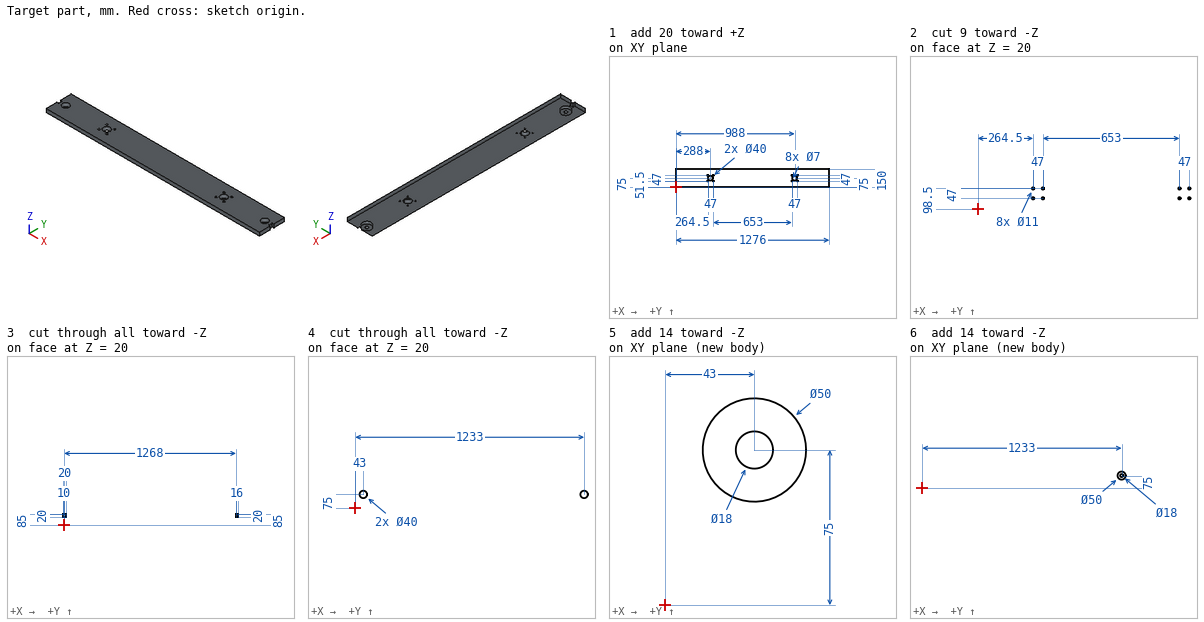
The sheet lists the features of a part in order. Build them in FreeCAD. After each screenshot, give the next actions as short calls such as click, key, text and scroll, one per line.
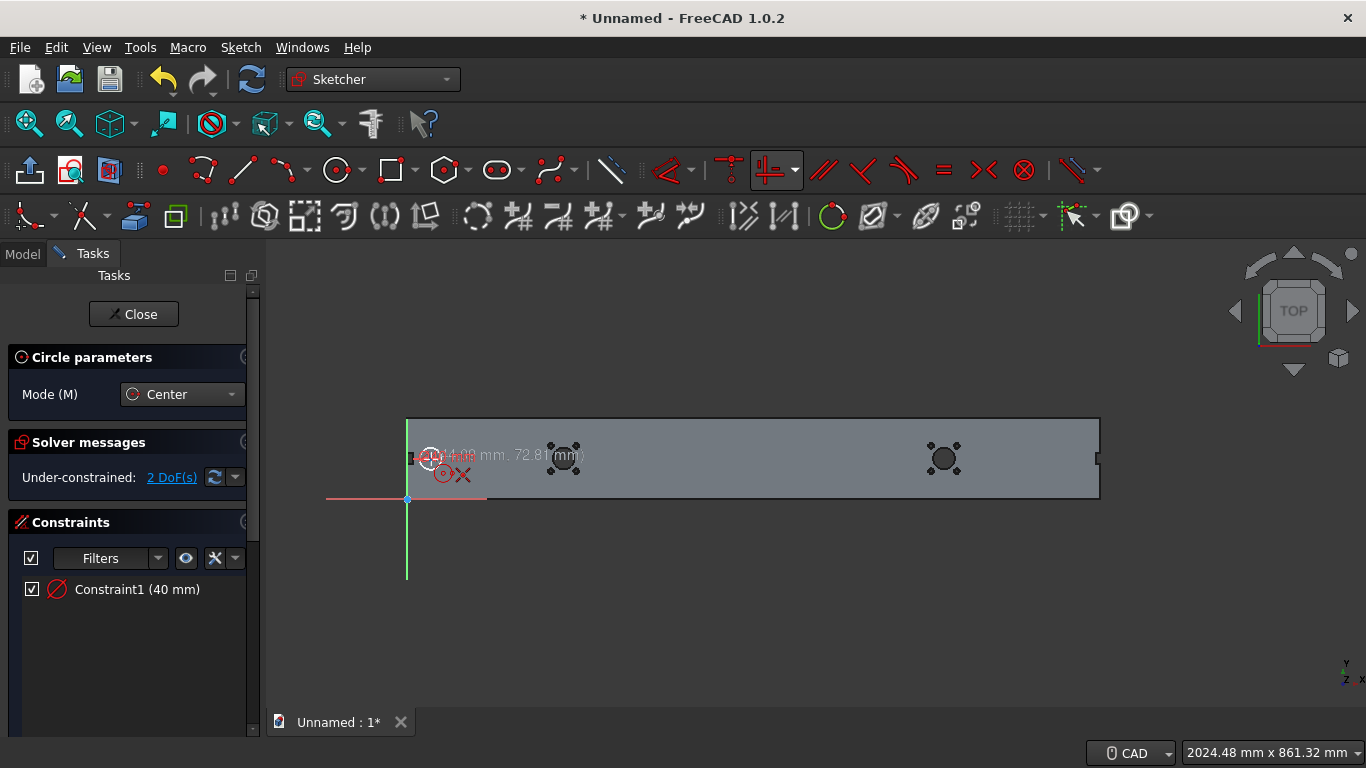
scroll(1077, 459, up, 4)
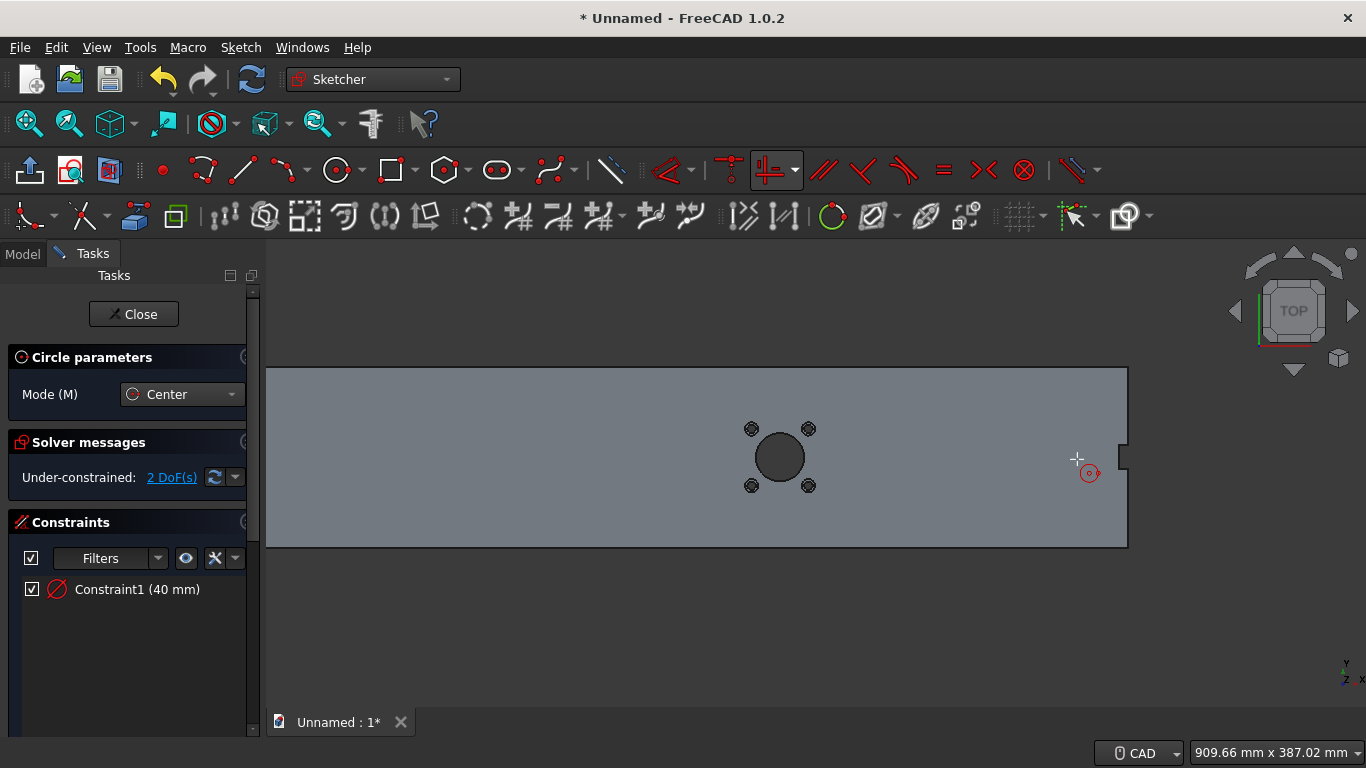
click(1076, 457)
move(1093, 440)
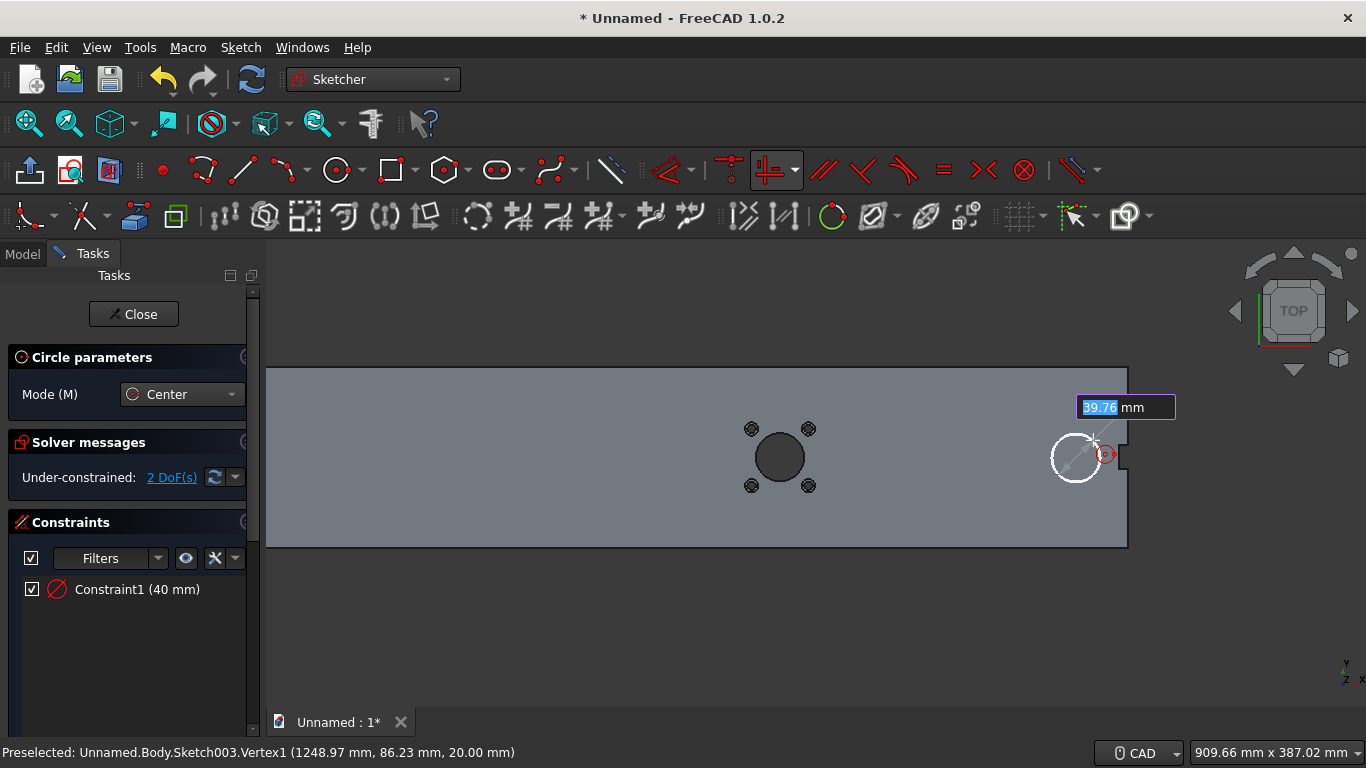
text(40)
key(Return)
key(Escape)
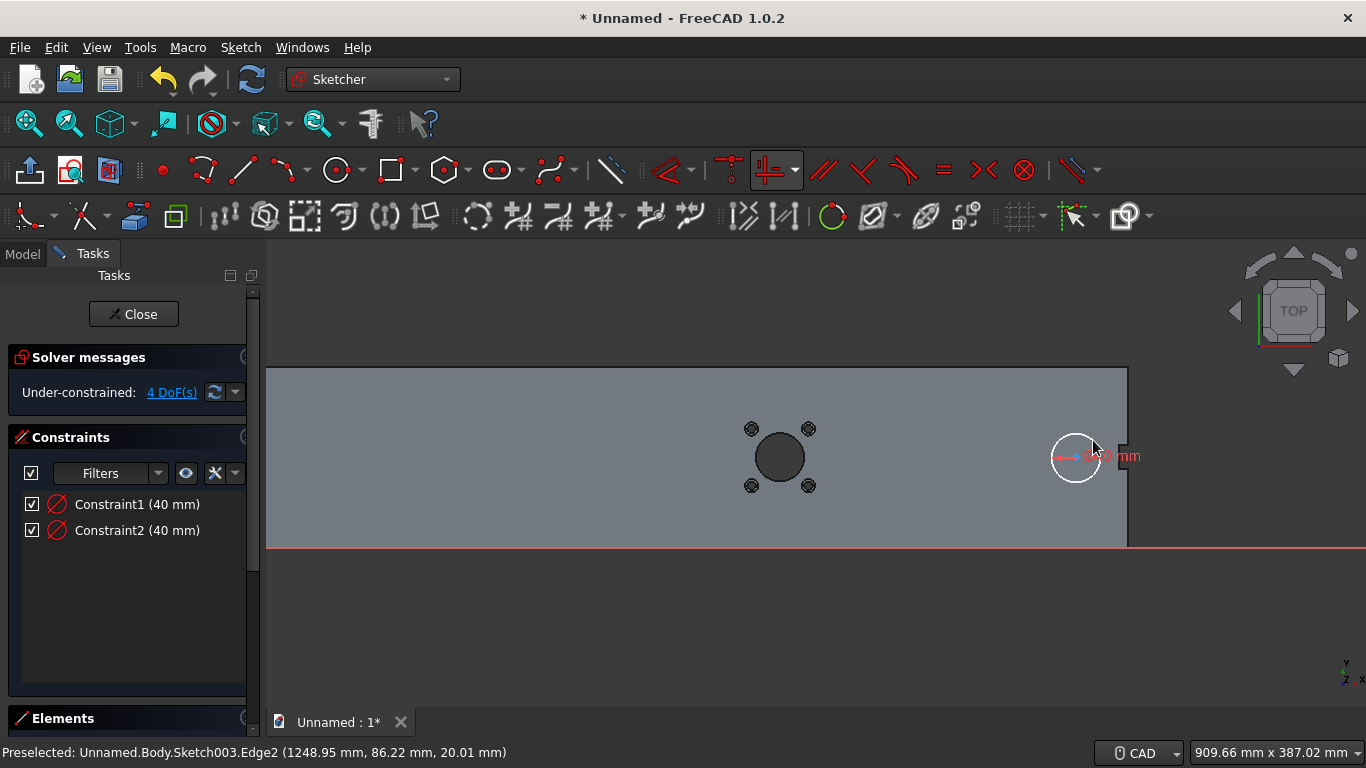
scroll(1078, 459, down, 4)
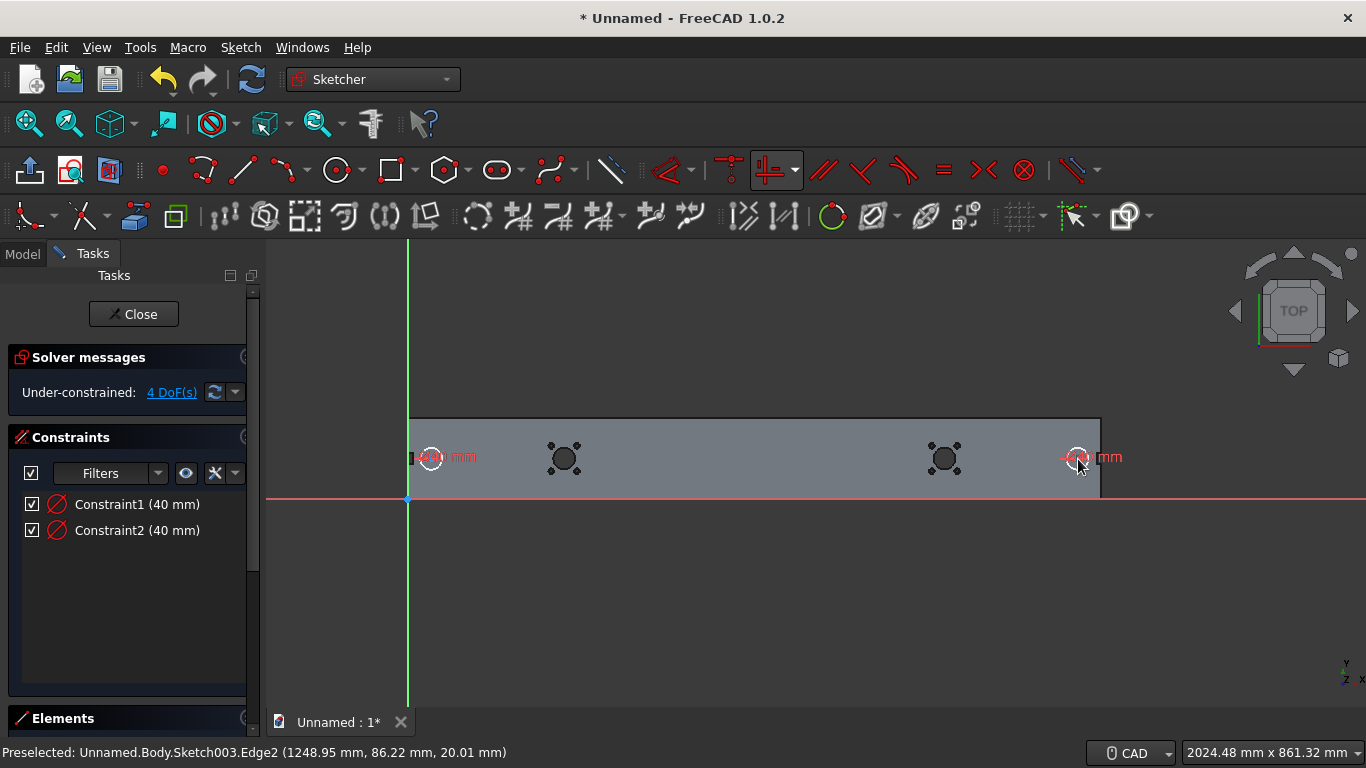
click(431, 459)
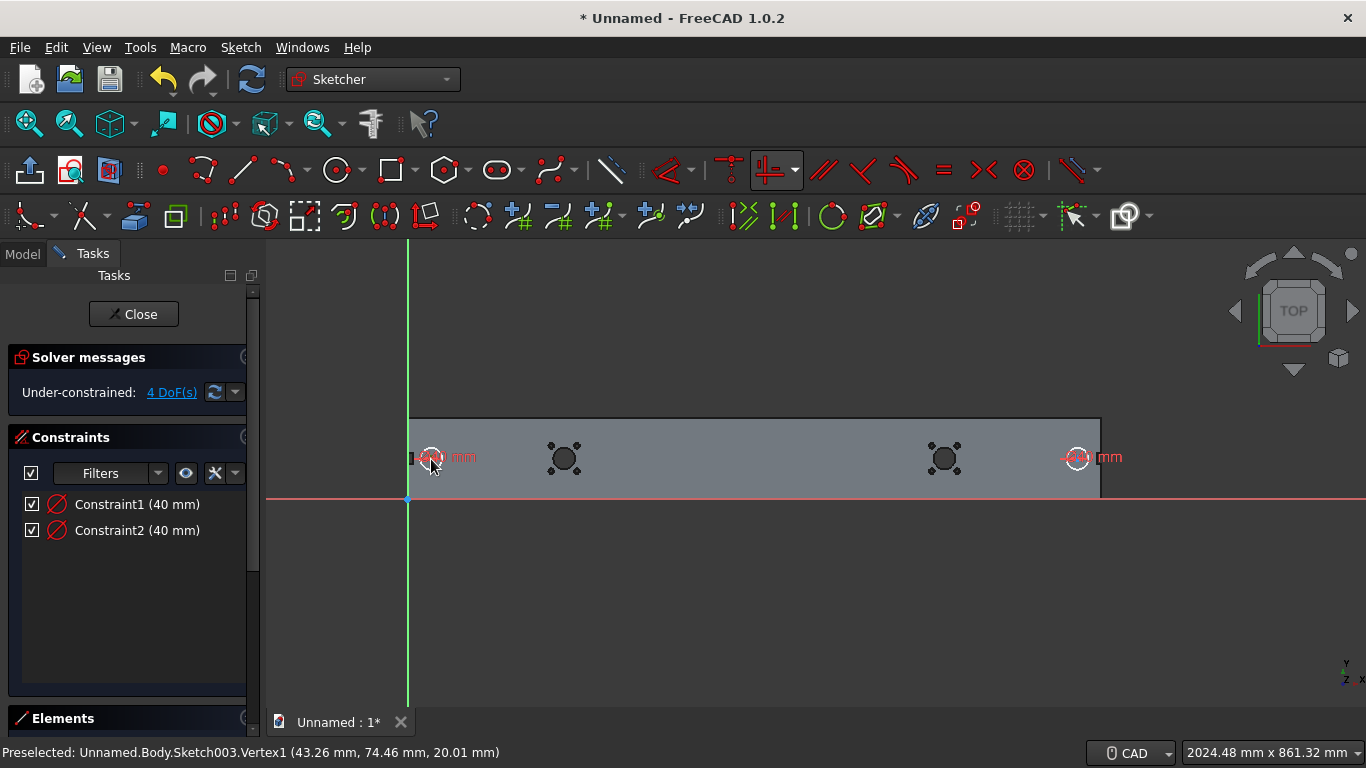
click(1078, 459)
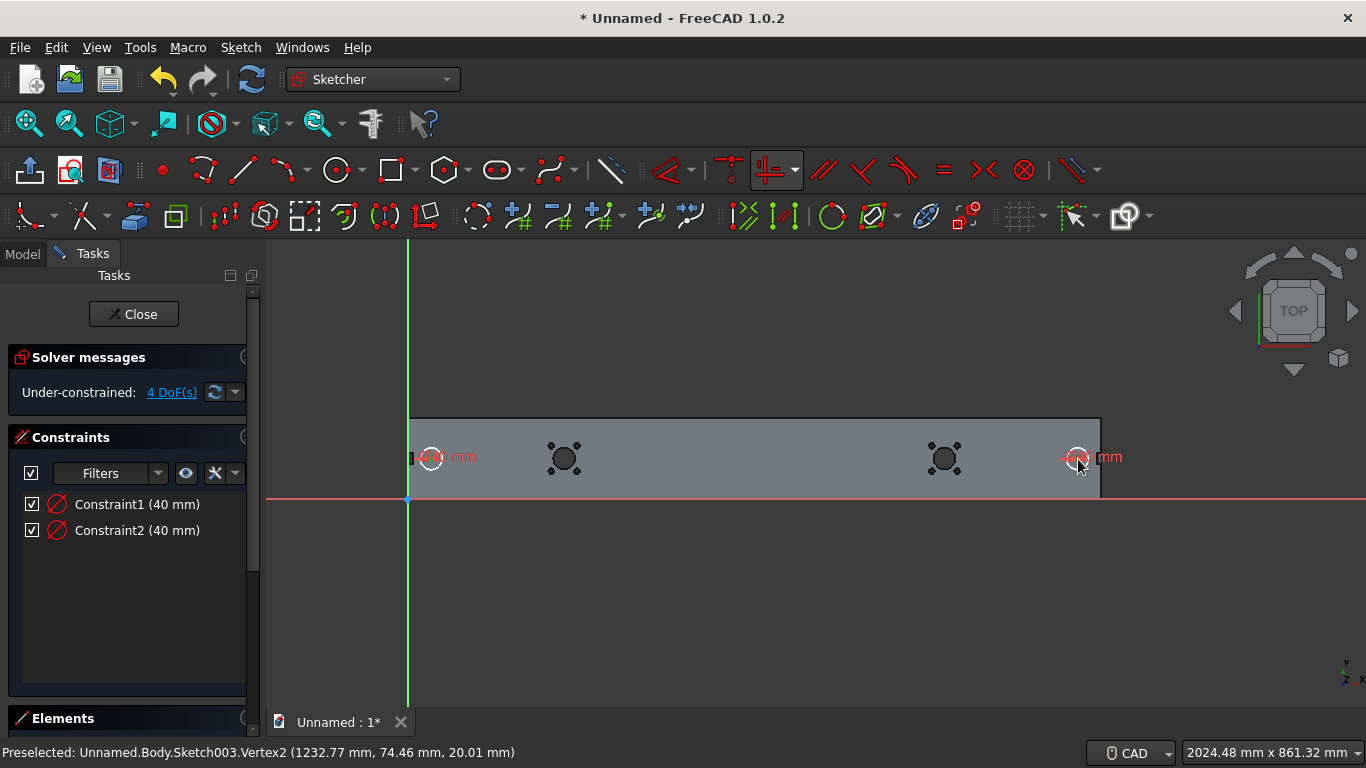
click(798, 170)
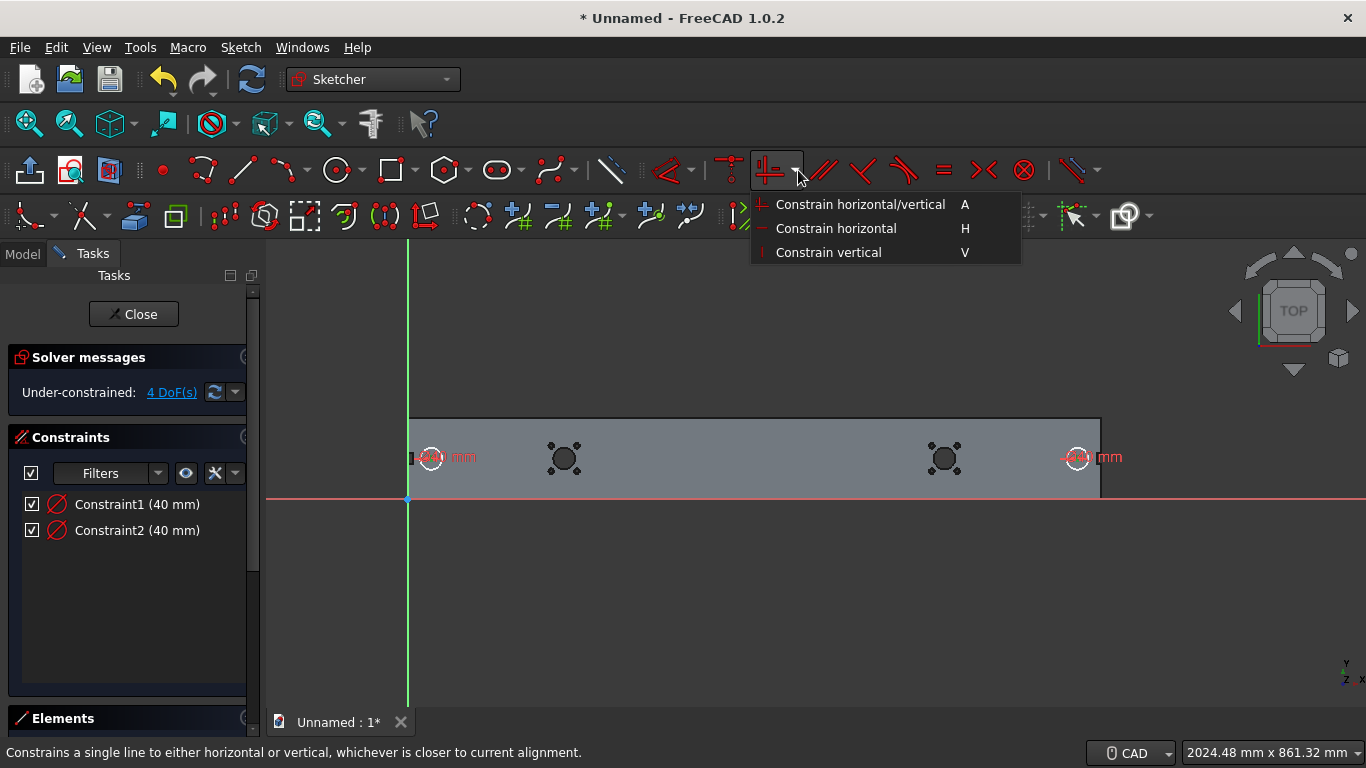
click(886, 228)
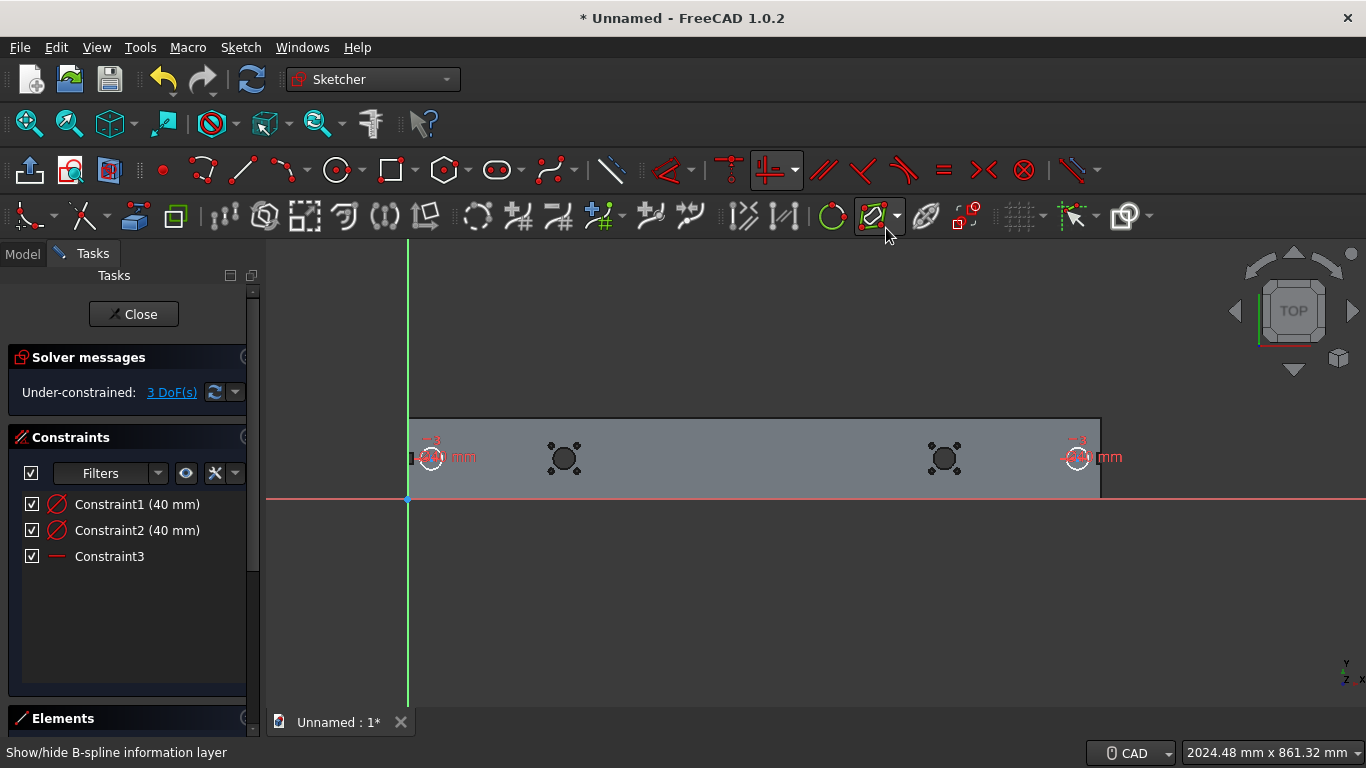
click(666, 170)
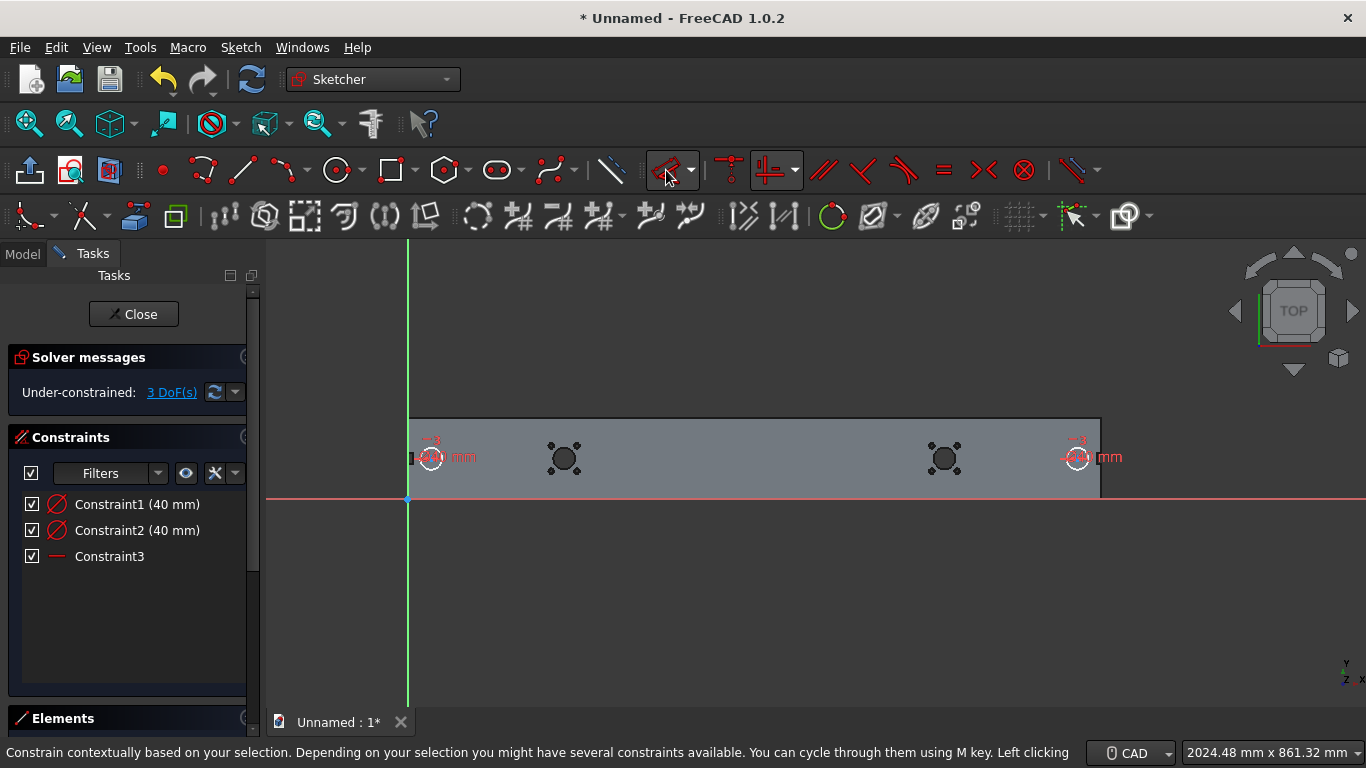
scroll(431, 459, up, 3)